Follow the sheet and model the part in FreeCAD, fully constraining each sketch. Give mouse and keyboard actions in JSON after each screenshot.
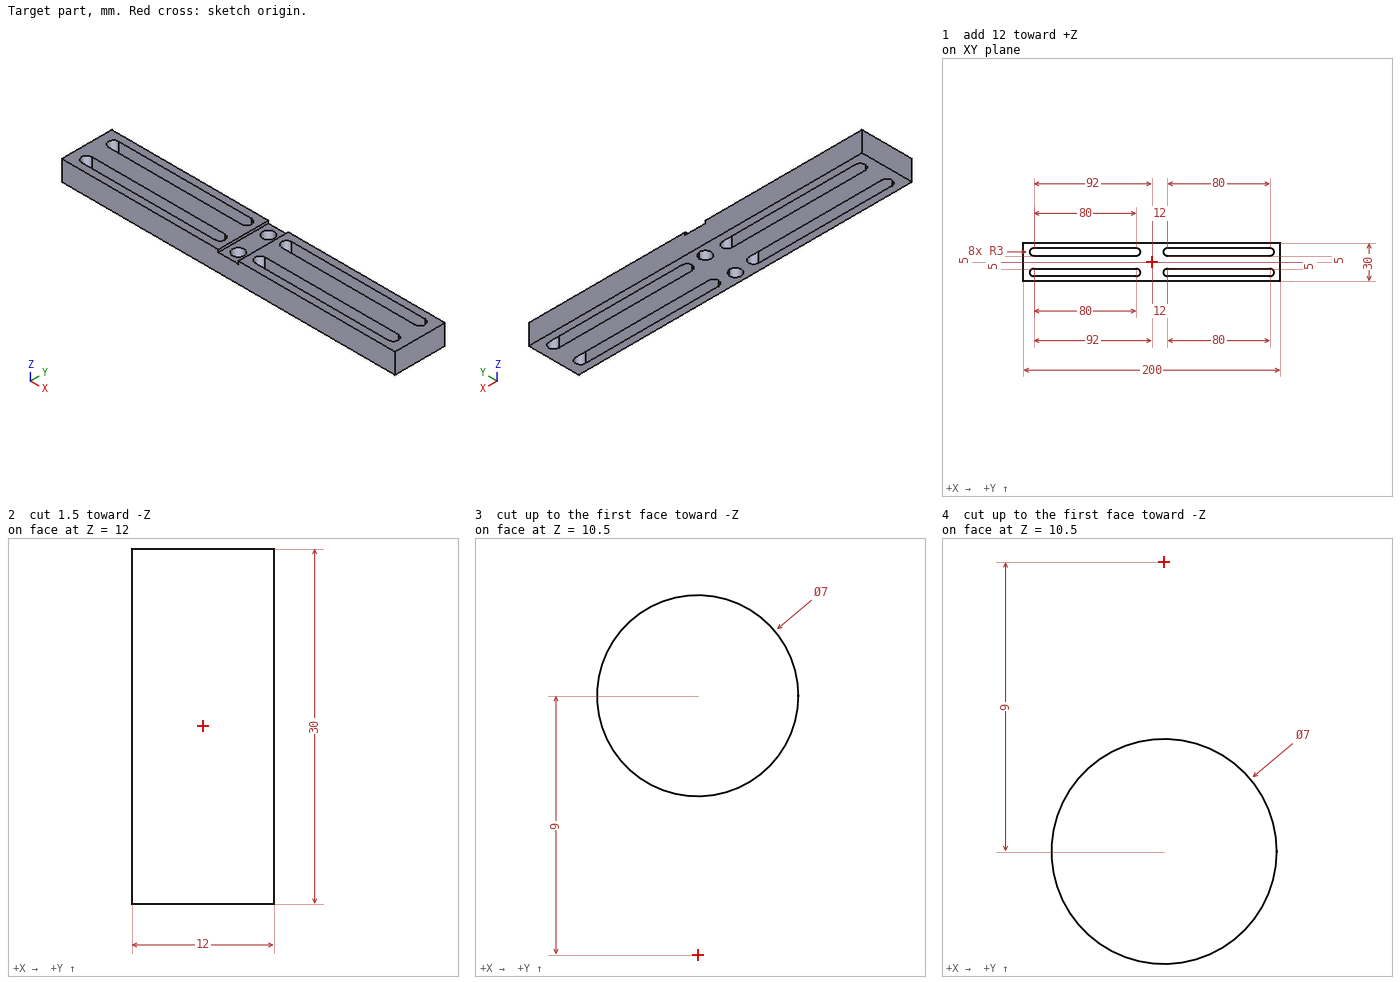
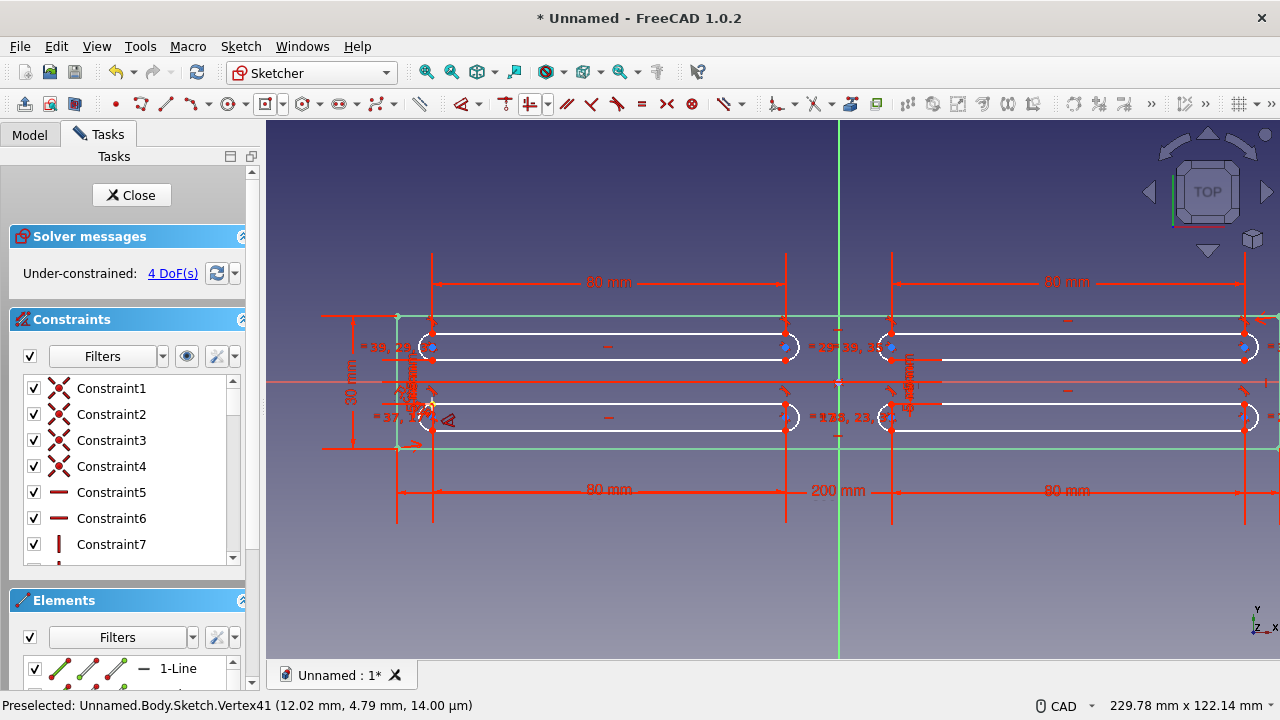
{"action": "left_click", "coordinate": [433, 404]}
{"action": "left_click", "coordinate": [636, 462]}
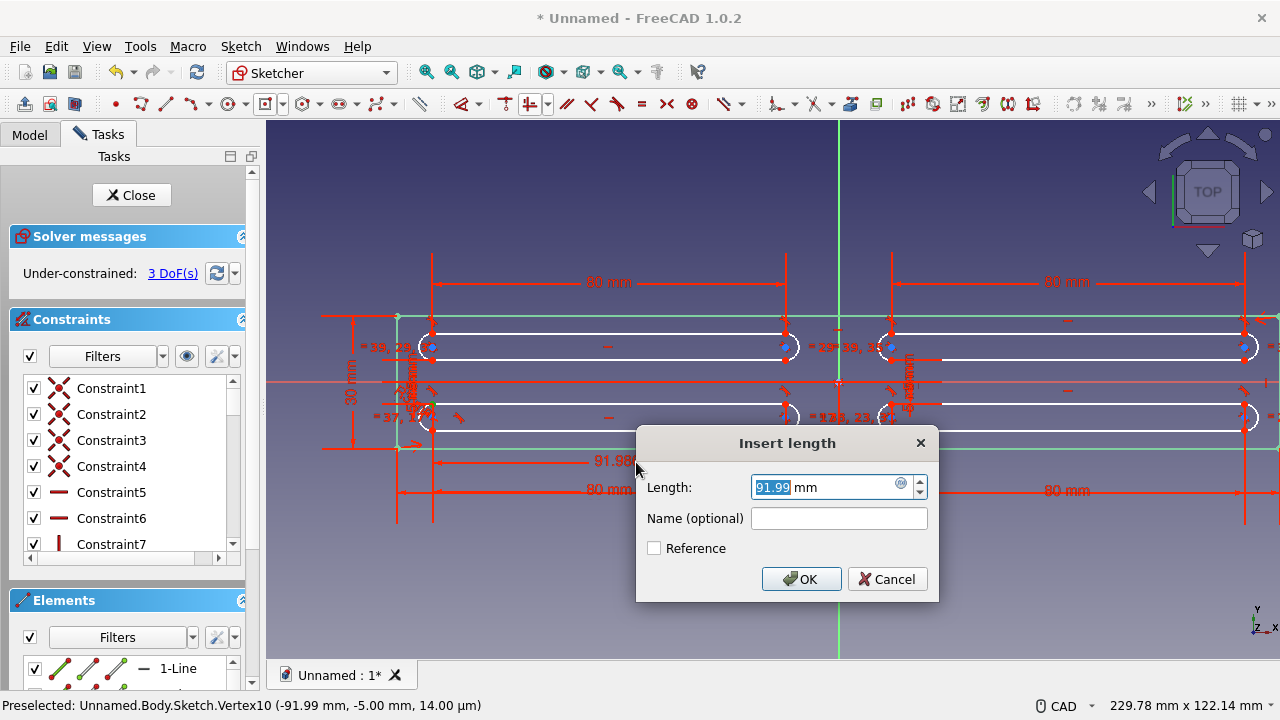
{"action": "type", "text": "92"}
{"action": "key", "text": "Return"}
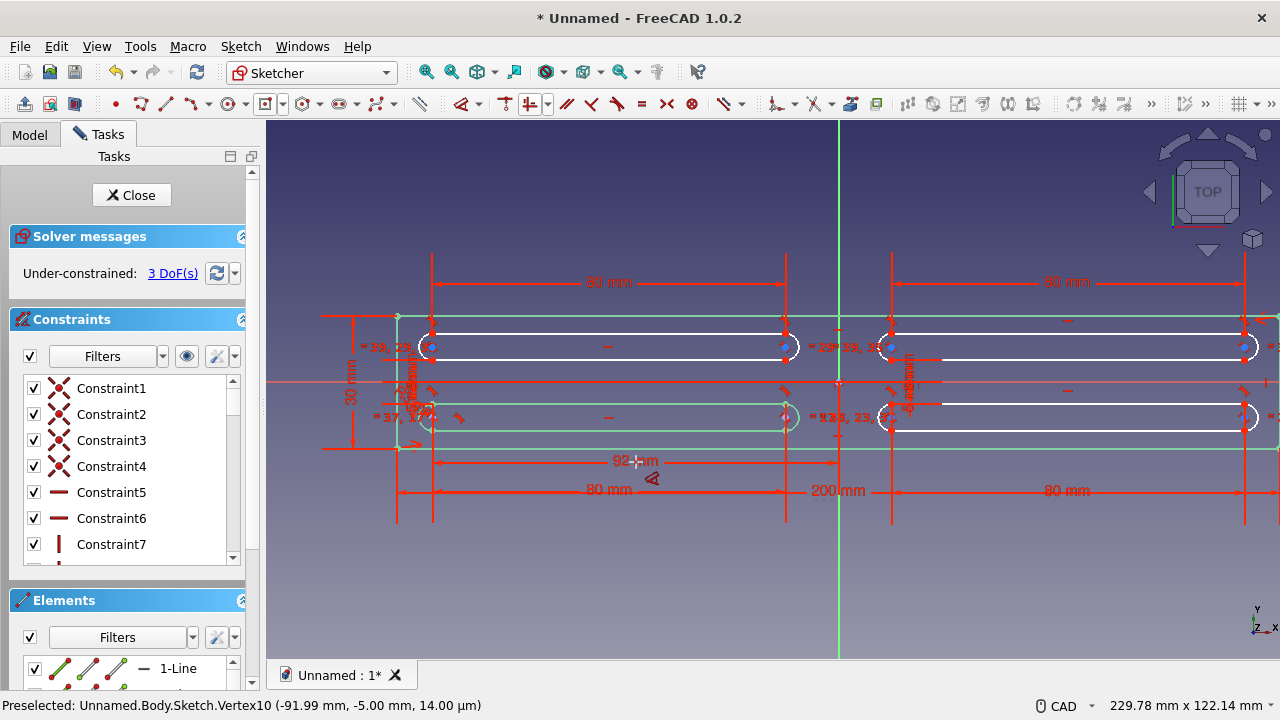
{"action": "left_click", "coordinate": [892, 404]}
{"action": "left_click", "coordinate": [865, 348]}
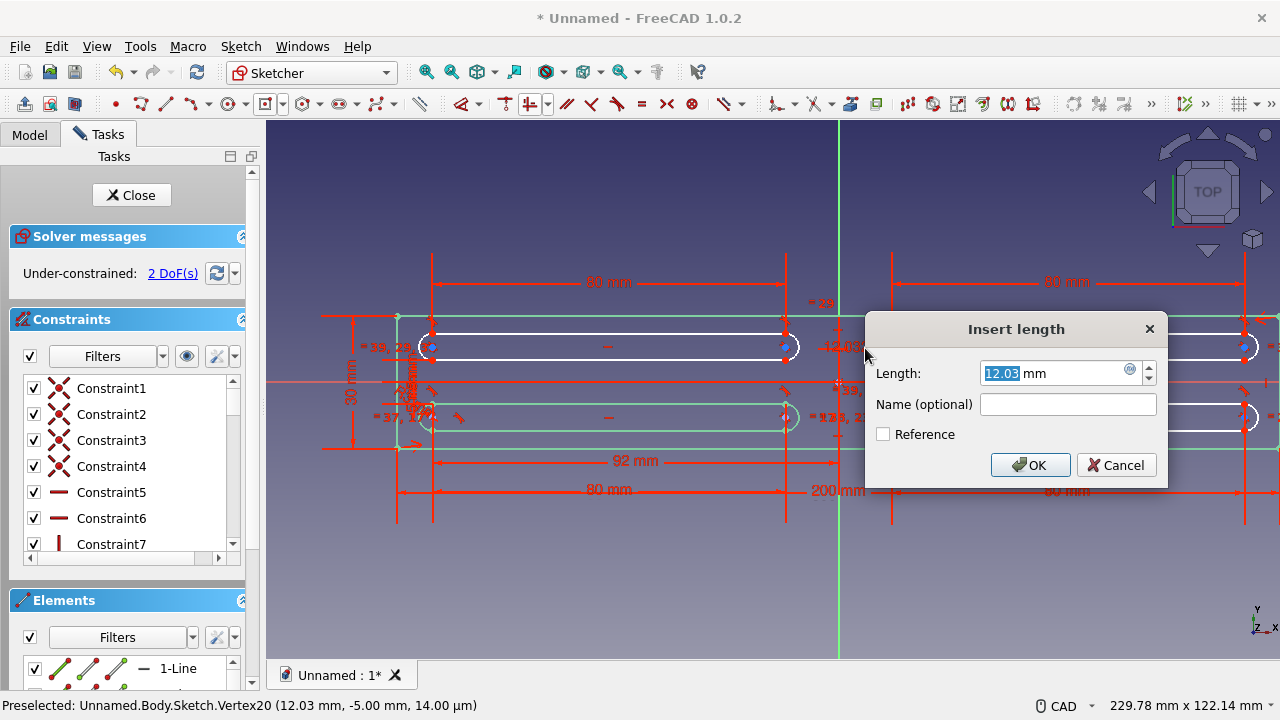
{"action": "type", "text": "12"}
{"action": "key", "text": "Return"}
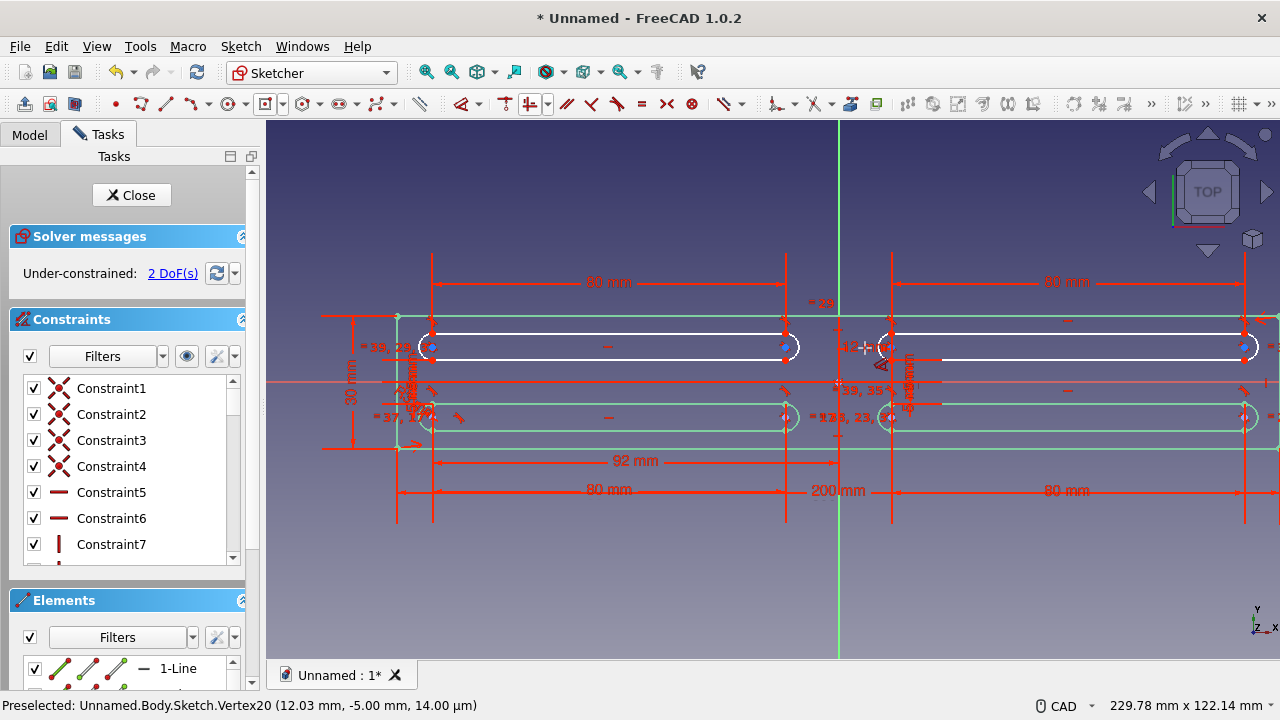
{"action": "left_click", "coordinate": [432, 334]}
{"action": "left_click", "coordinate": [729, 300]}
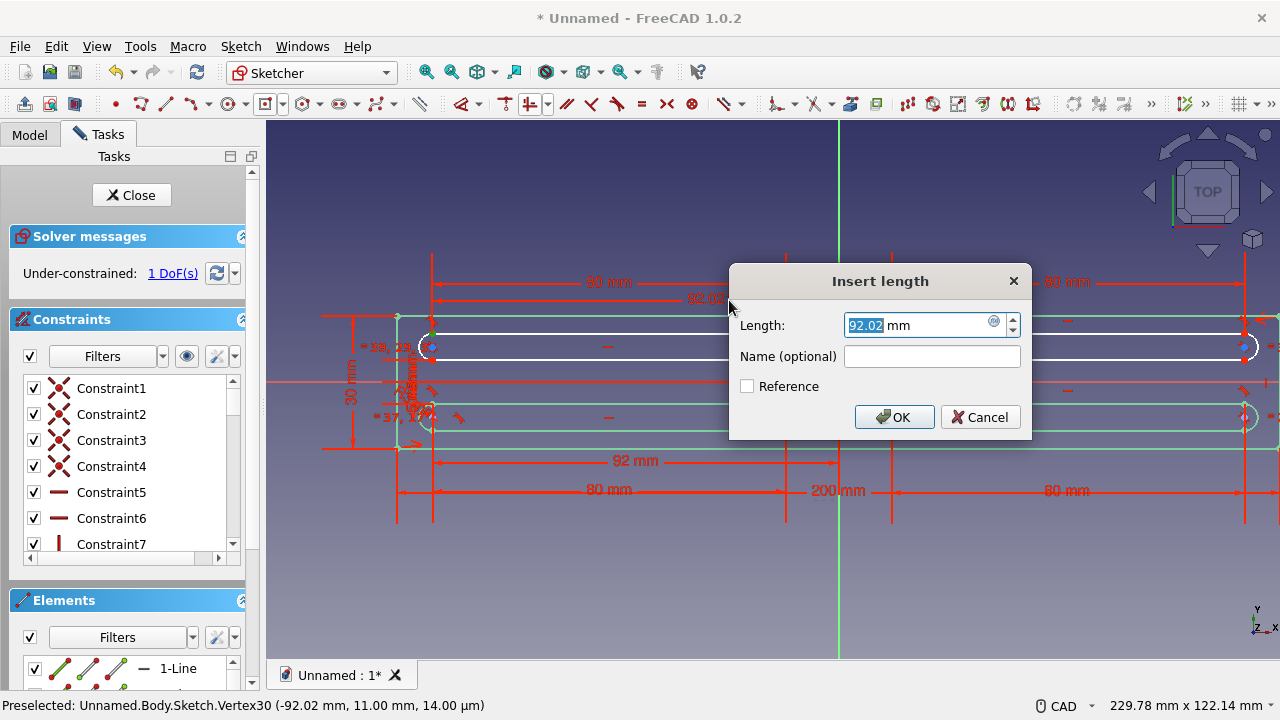
{"action": "type", "text": "92"}
{"action": "key", "text": "Return"}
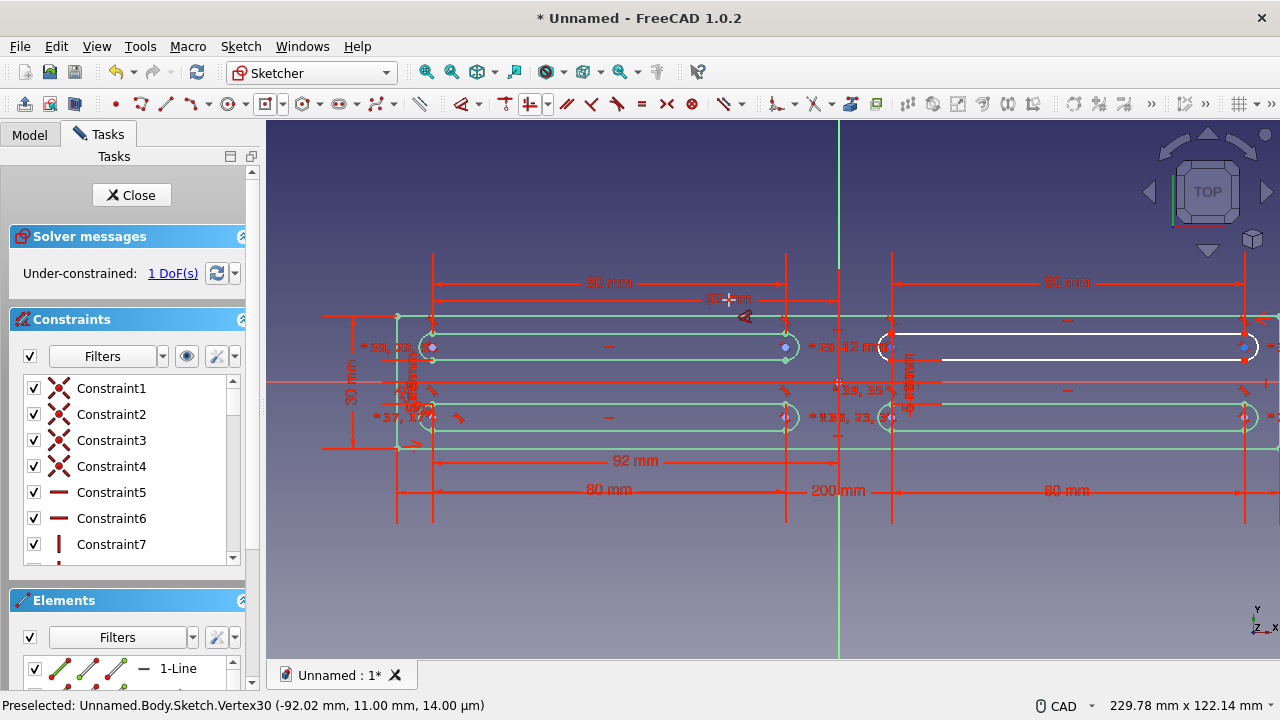
{"action": "left_click", "coordinate": [892, 334]}
{"action": "left_click", "coordinate": [865, 300]}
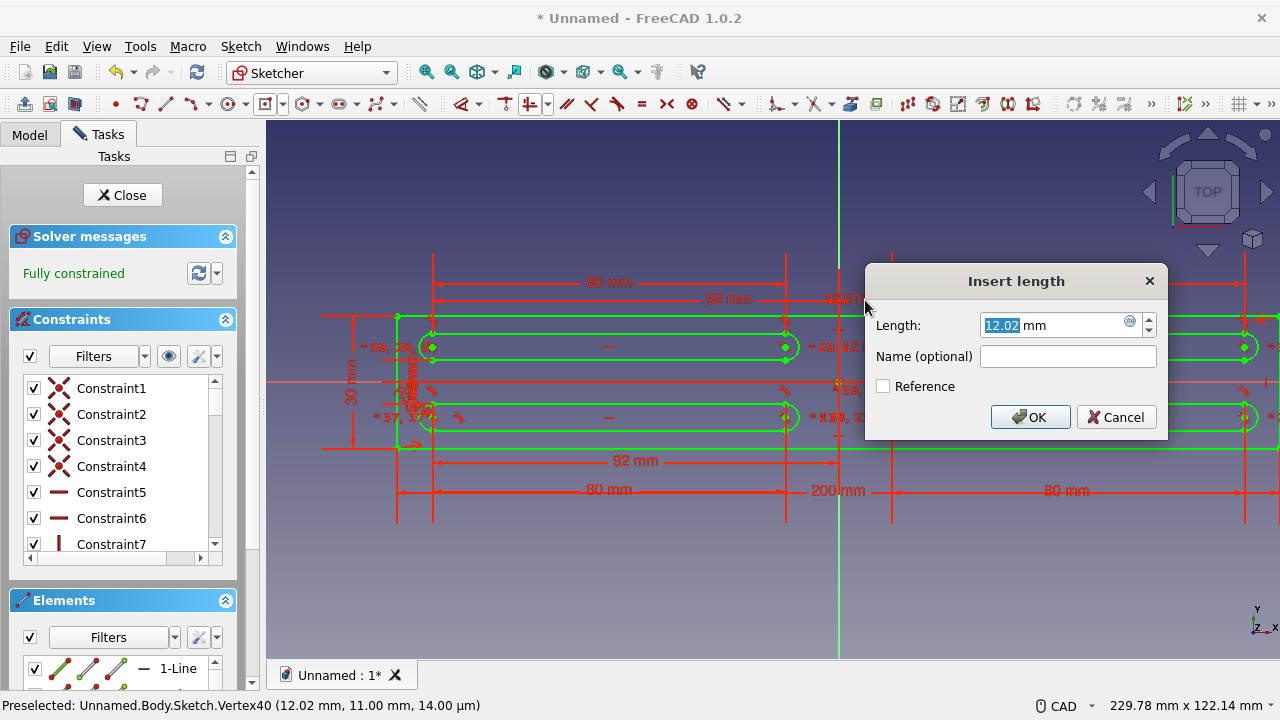
{"action": "type", "text": "12"}
{"action": "key", "text": "Return"}
{"action": "key", "text": "Escape"}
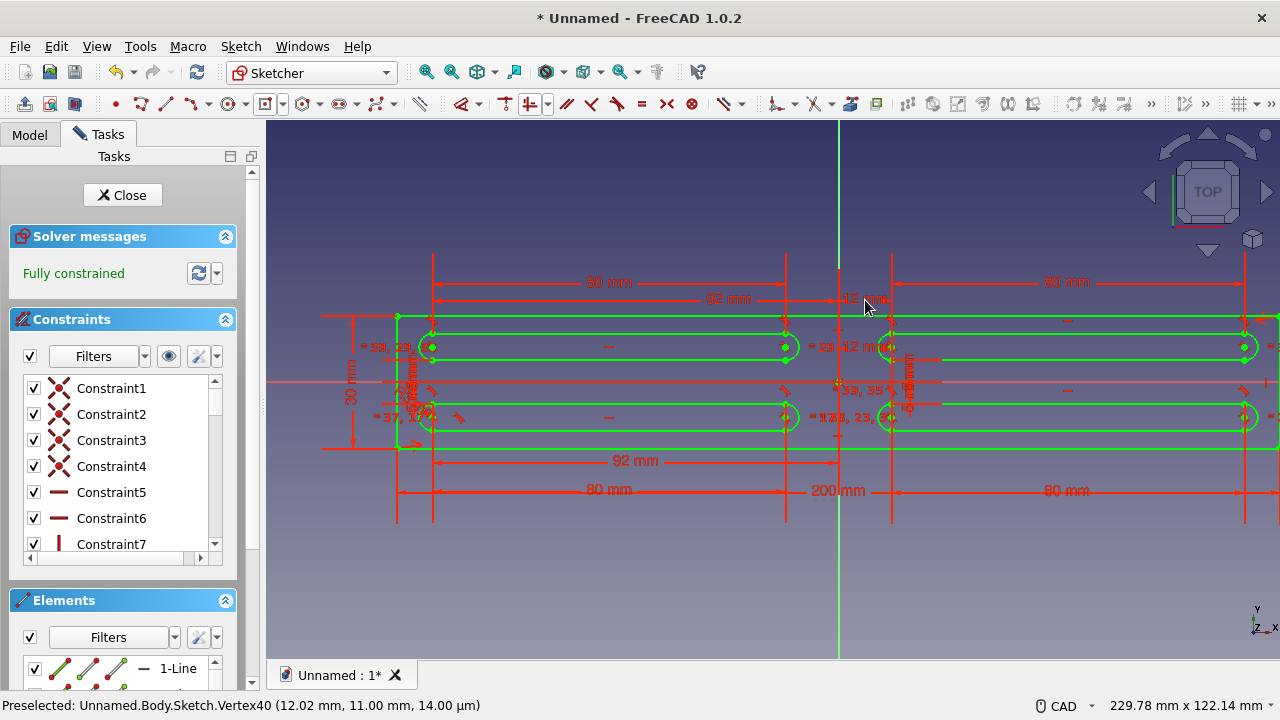
{"action": "left_click", "coordinate": [123, 195]}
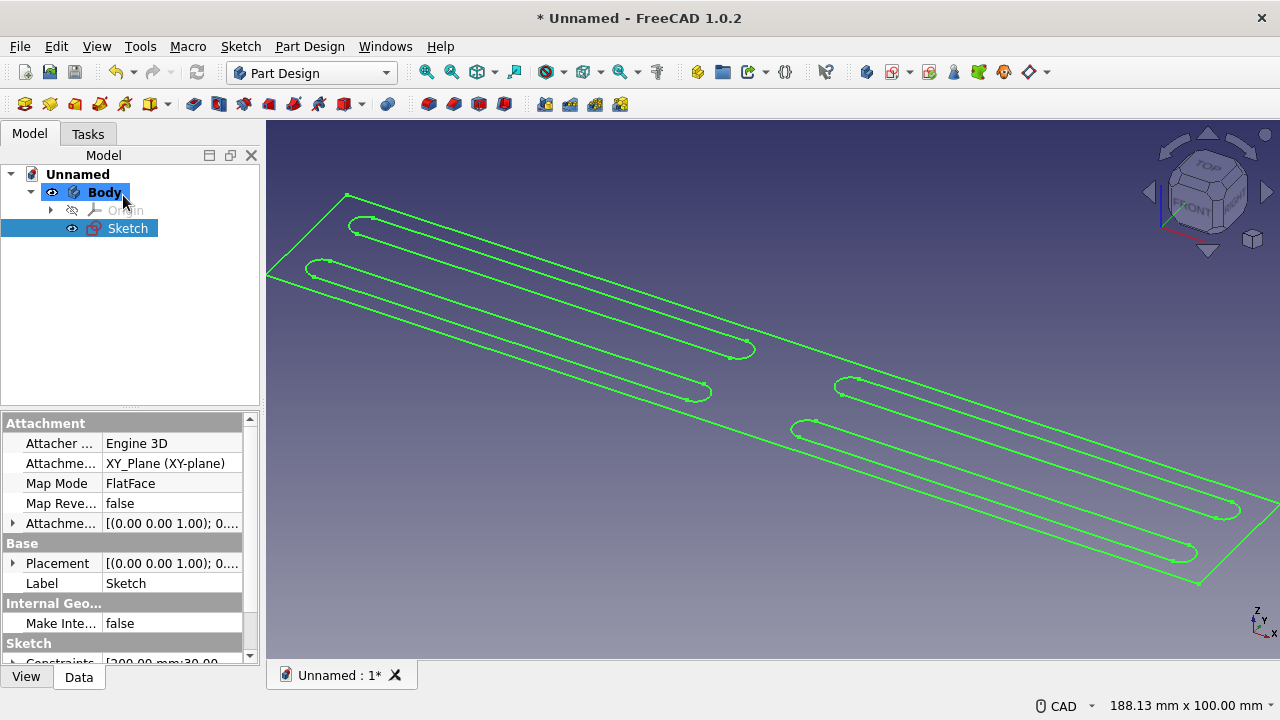
{"action": "left_click", "coordinate": [25, 104]}